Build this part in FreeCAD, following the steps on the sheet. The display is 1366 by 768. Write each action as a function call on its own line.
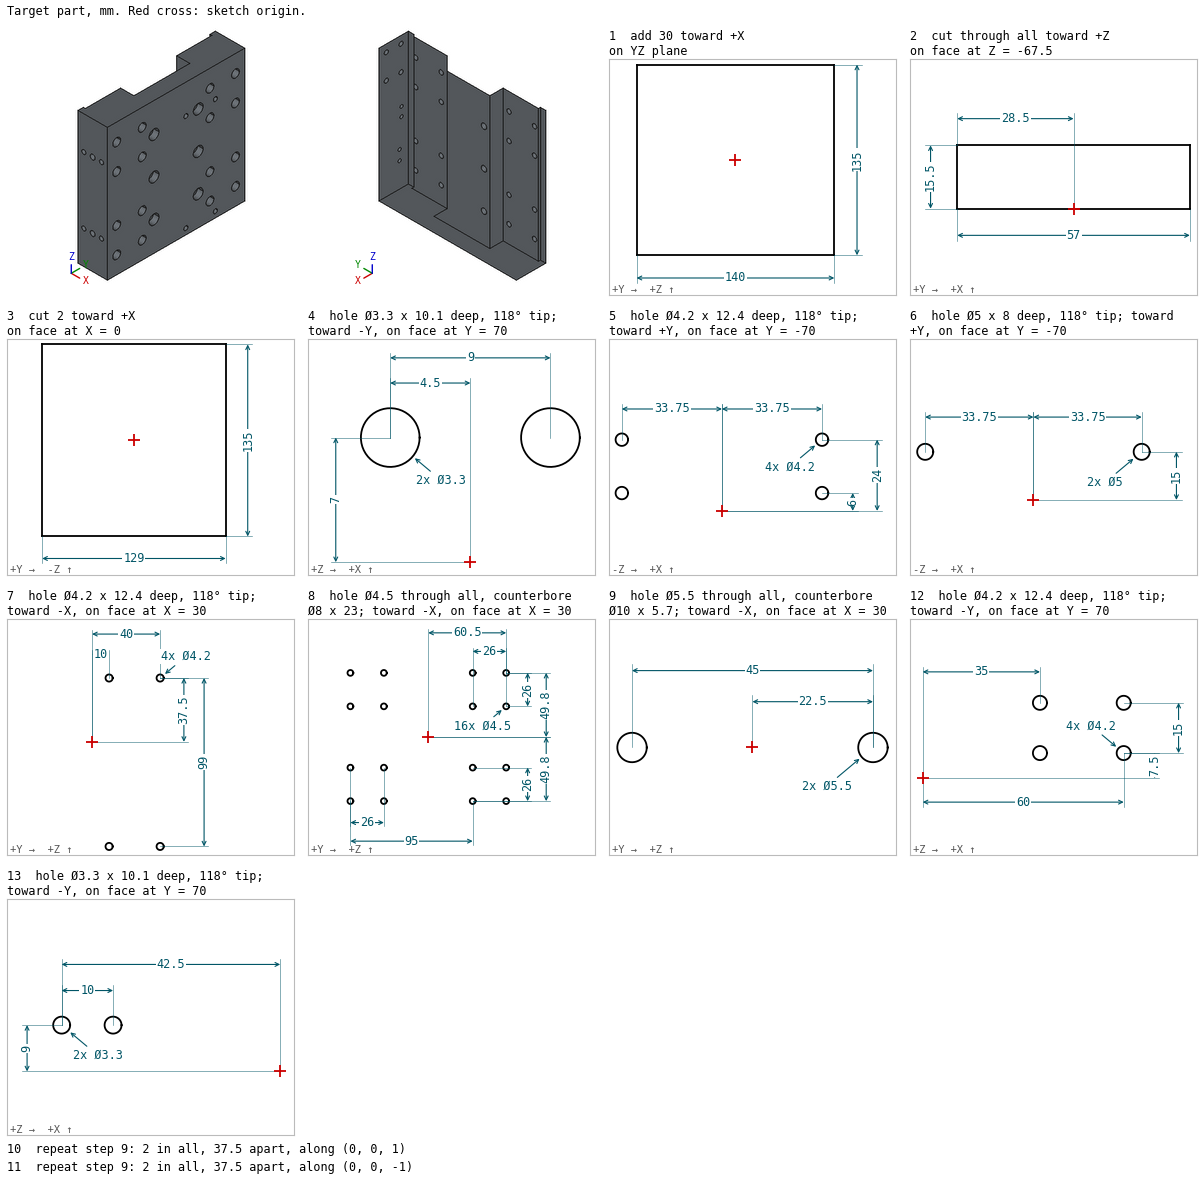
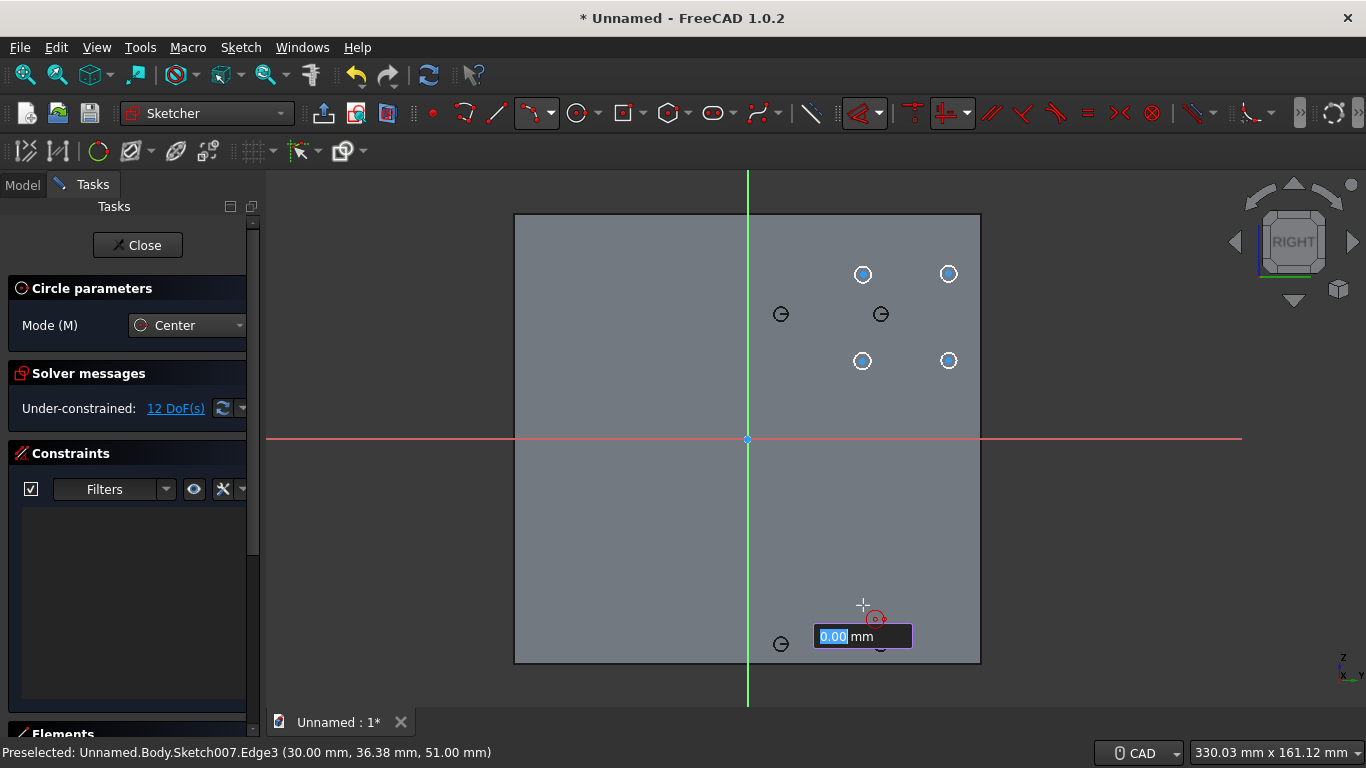
scroll(868, 600, up, 4)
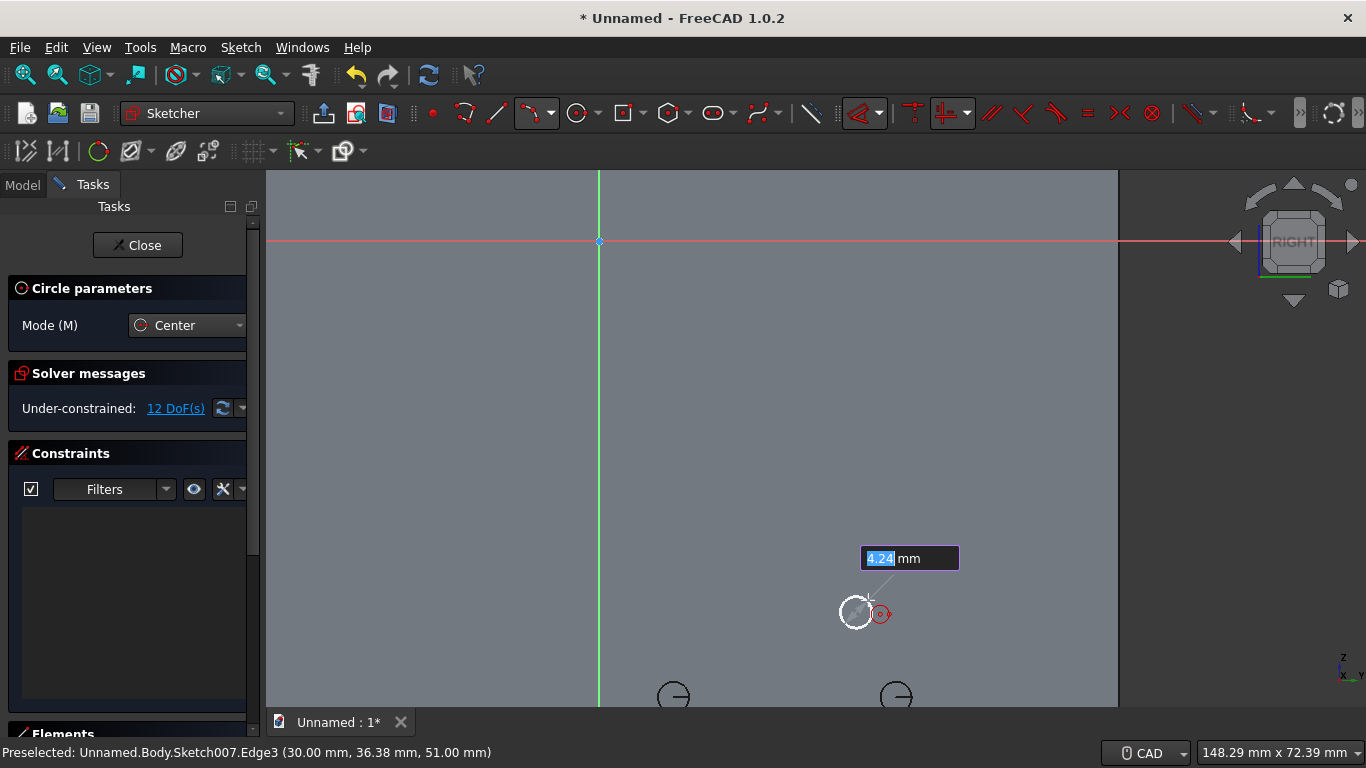
click(867, 599)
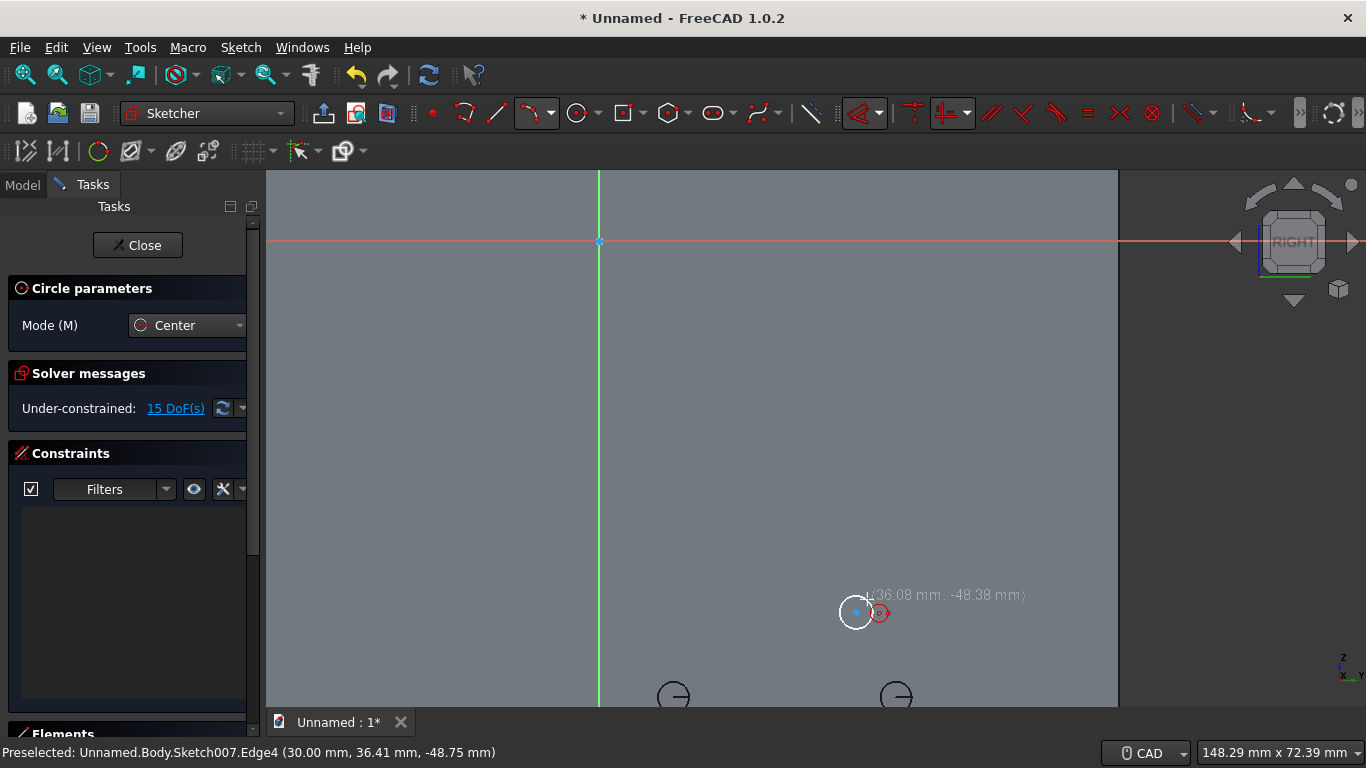
scroll(855, 418, up, 2)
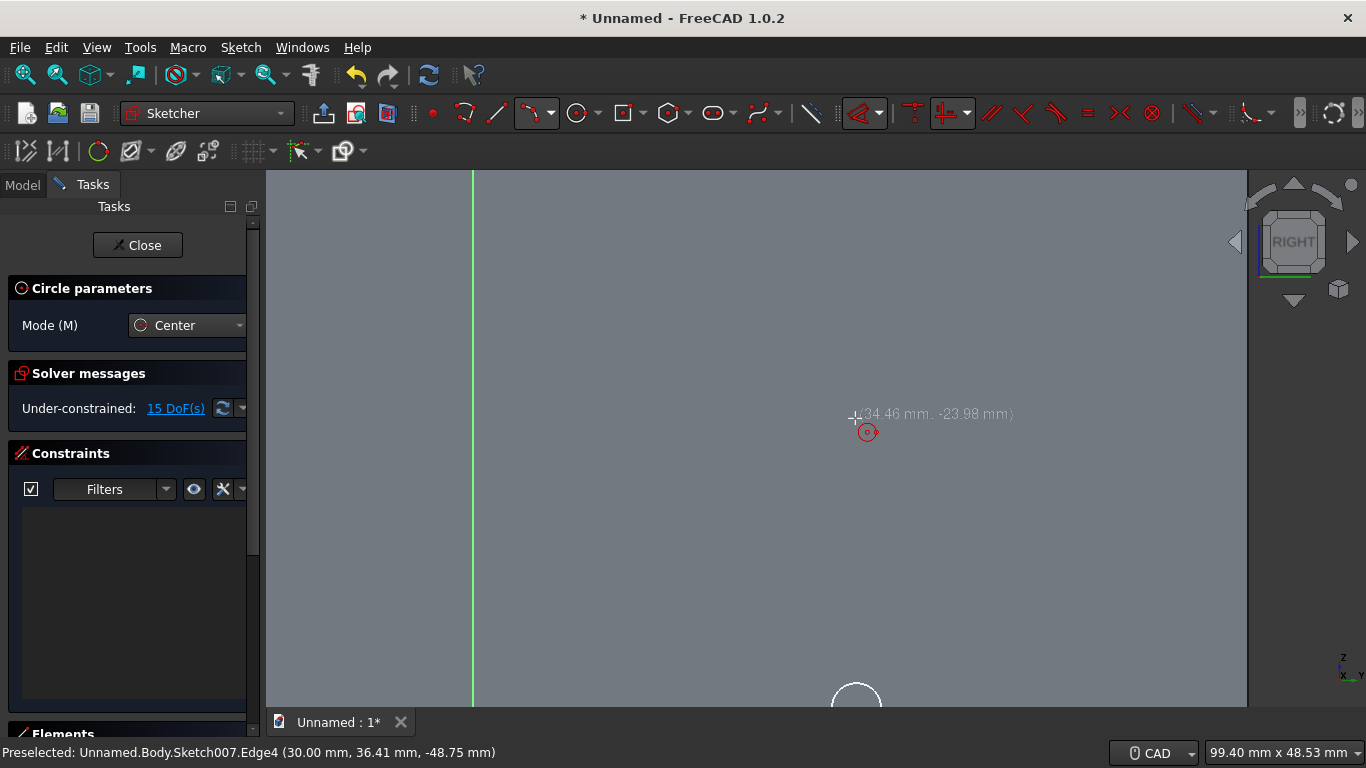
scroll(866, 561, down, 6)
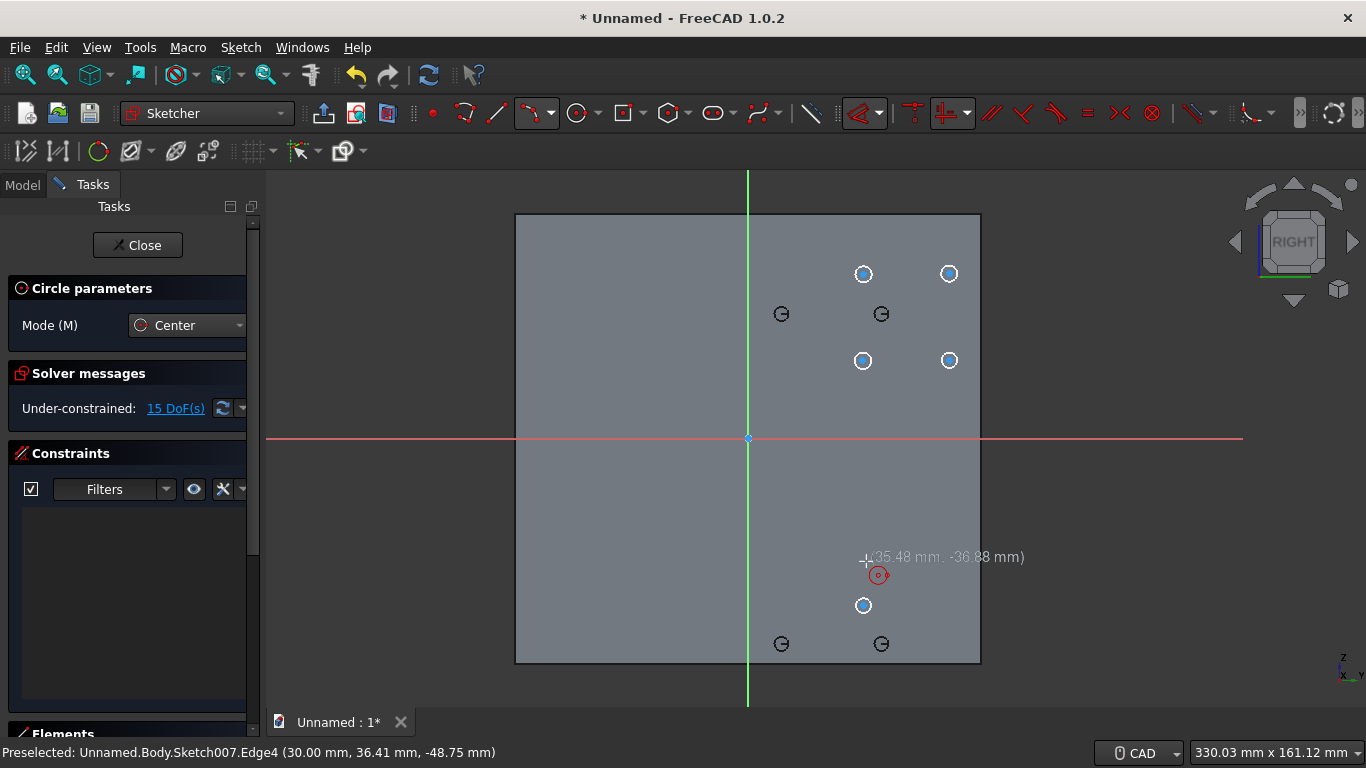
click(863, 518)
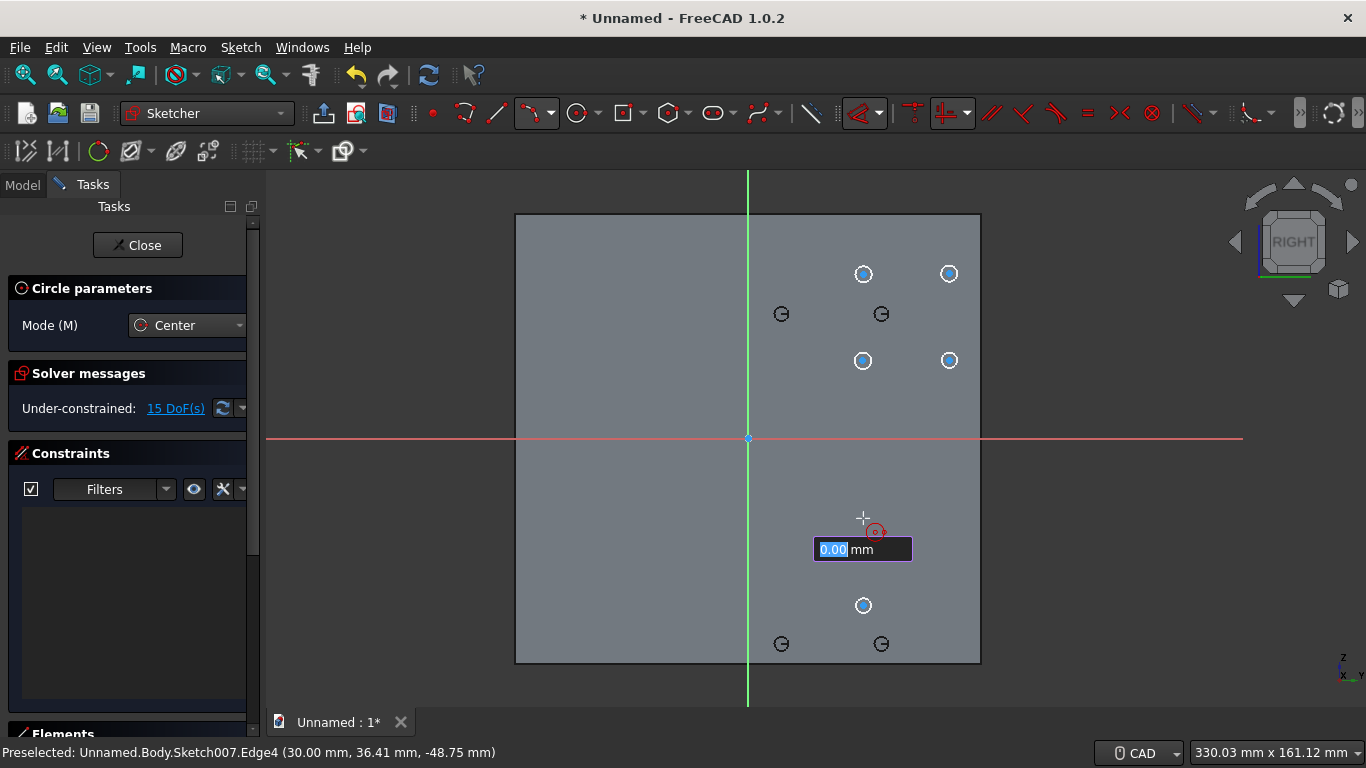
scroll(868, 513, up, 4)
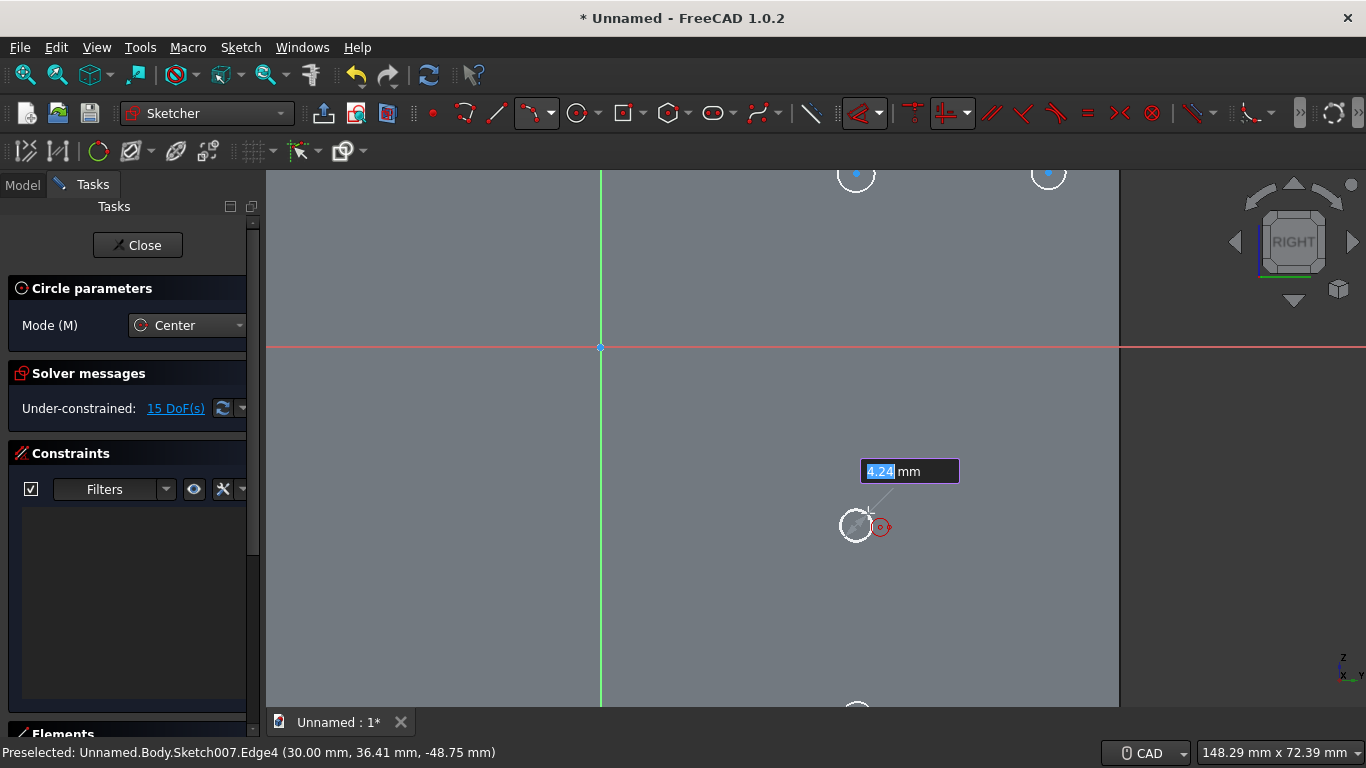
click(868, 512)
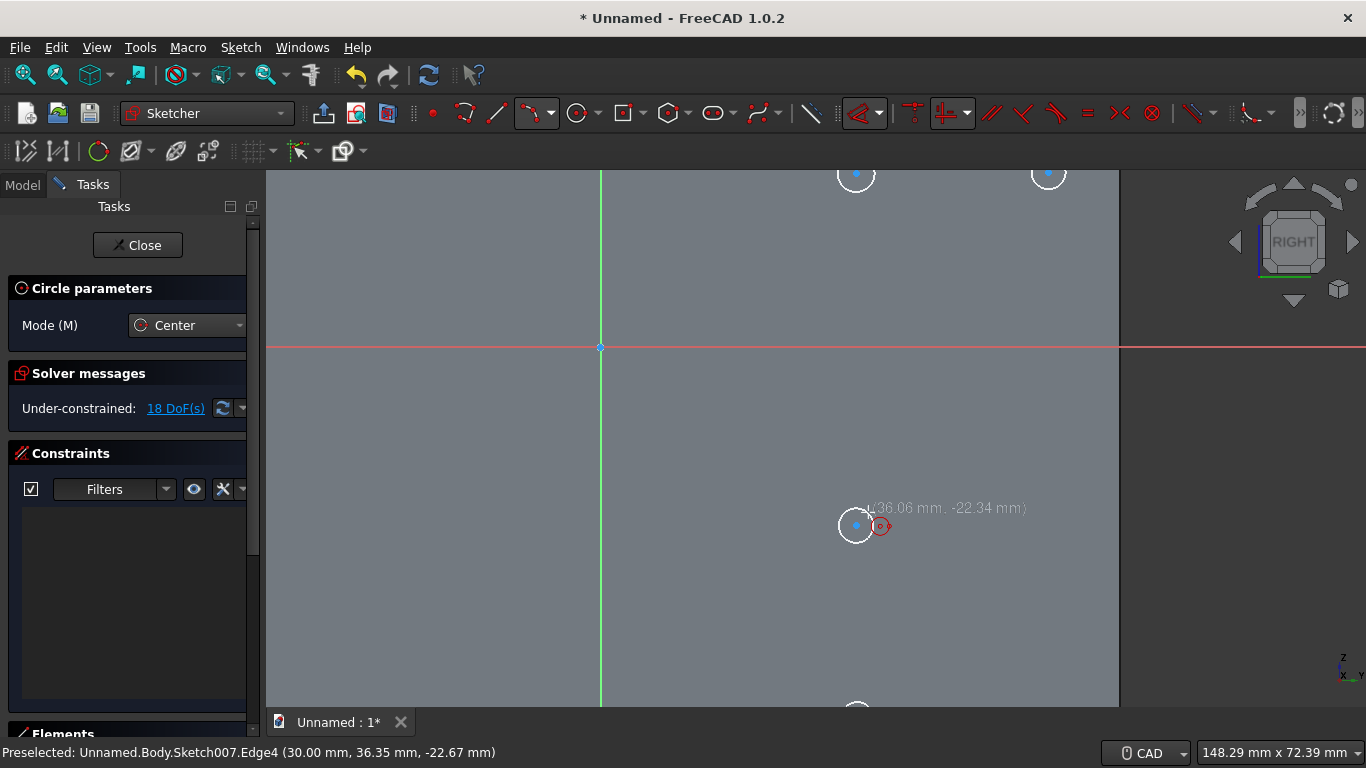
scroll(1049, 524, up, 2)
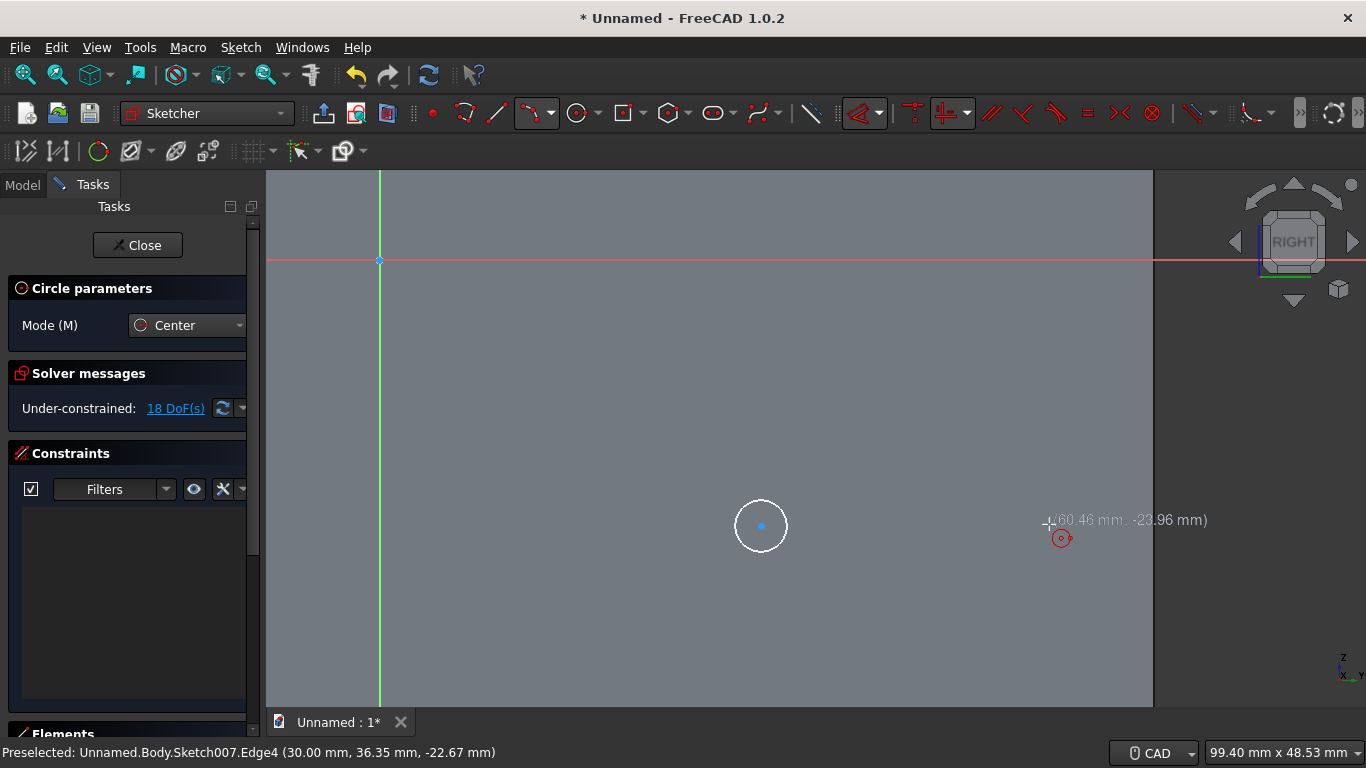
scroll(906, 515, down, 6)